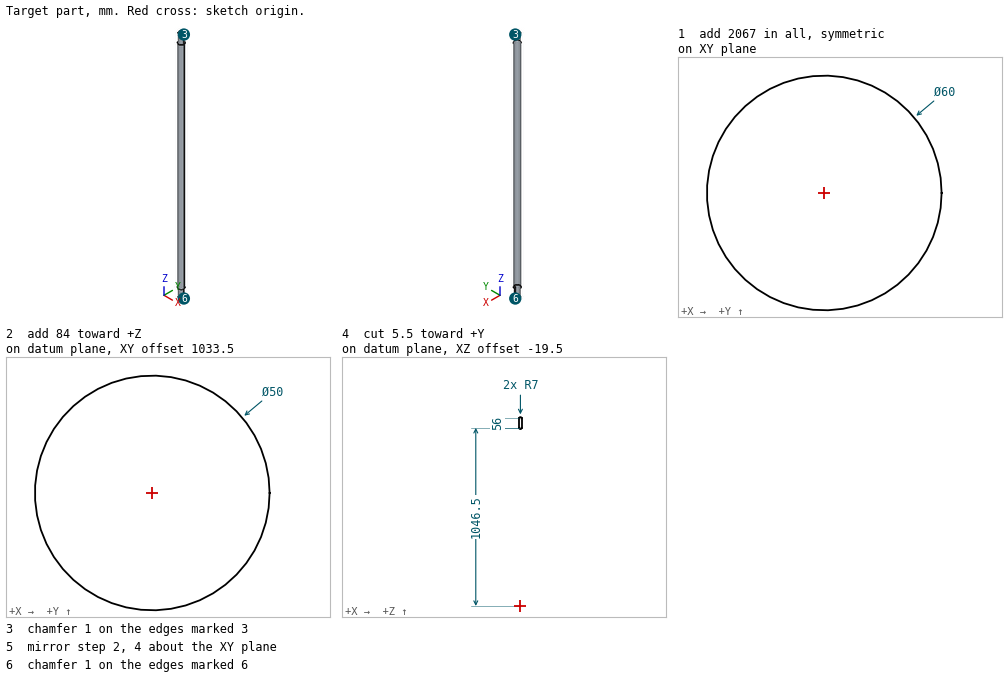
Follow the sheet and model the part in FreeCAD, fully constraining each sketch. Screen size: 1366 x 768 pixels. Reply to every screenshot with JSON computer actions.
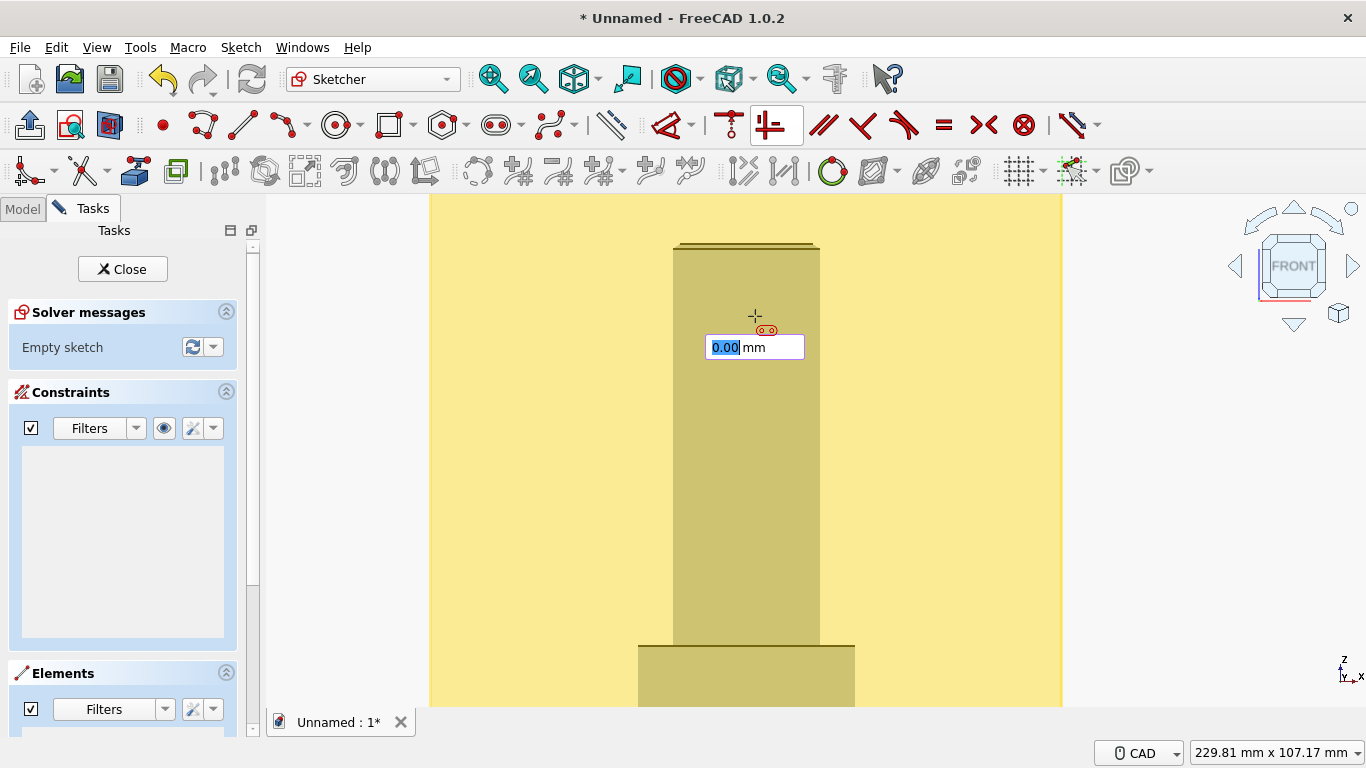
{"action": "left_click", "coordinate": [713, 450]}
{"action": "key", "text": "Escape"}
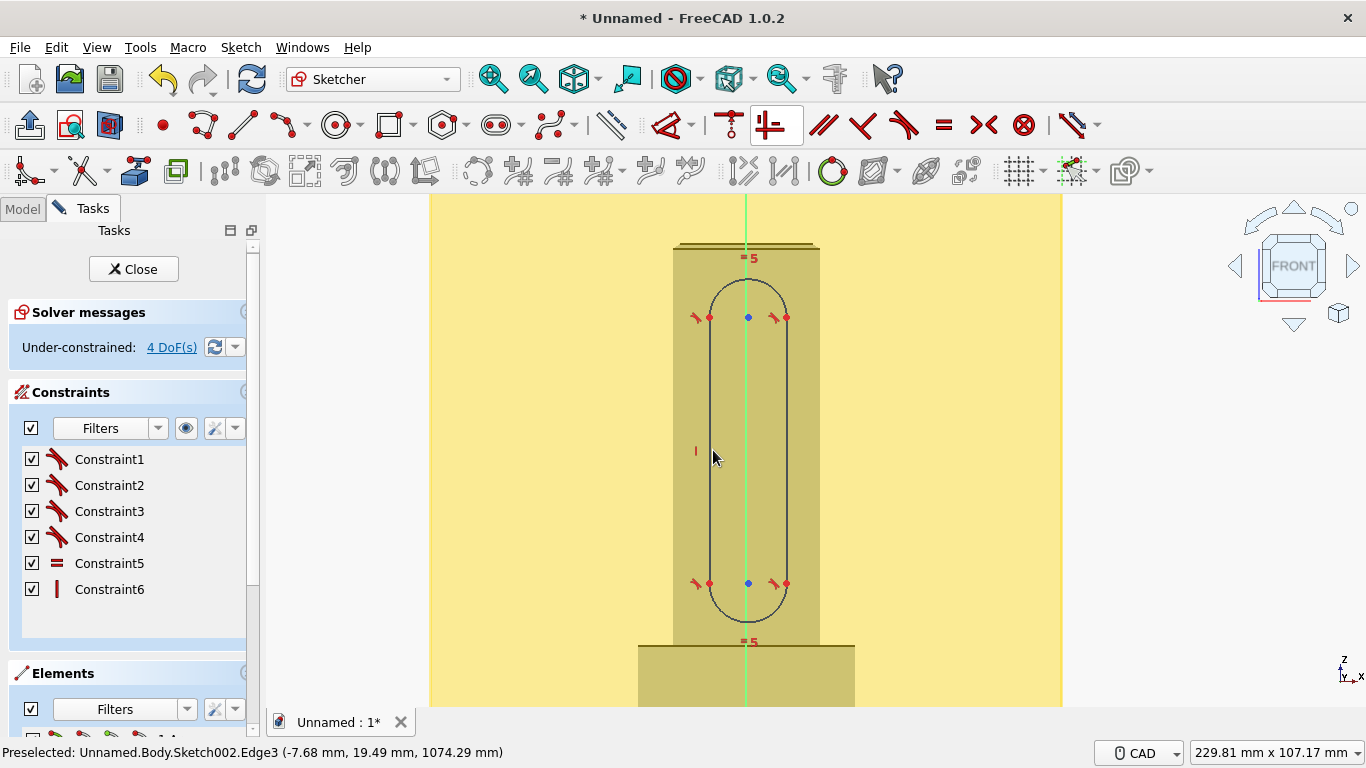
{"action": "left_click", "coordinate": [748, 584]}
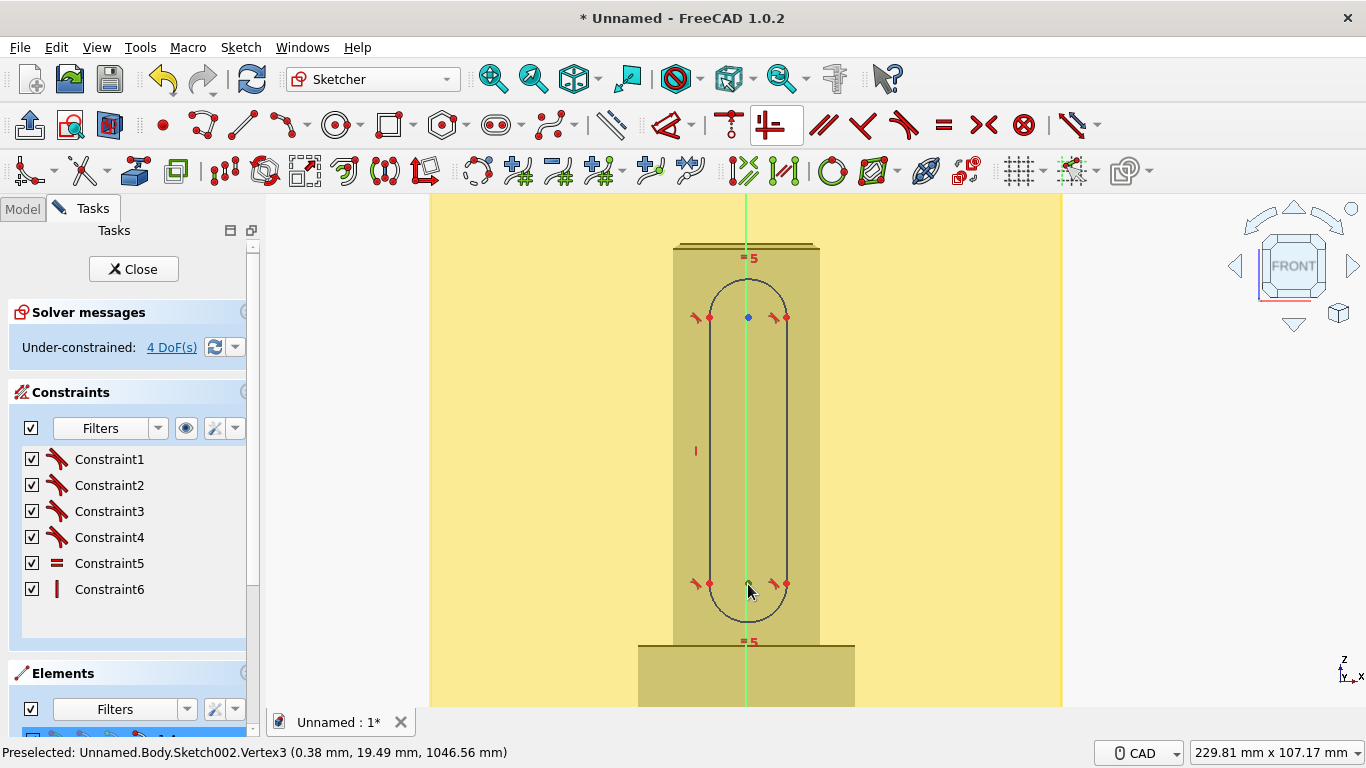
{"action": "left_click", "coordinate": [746, 548]}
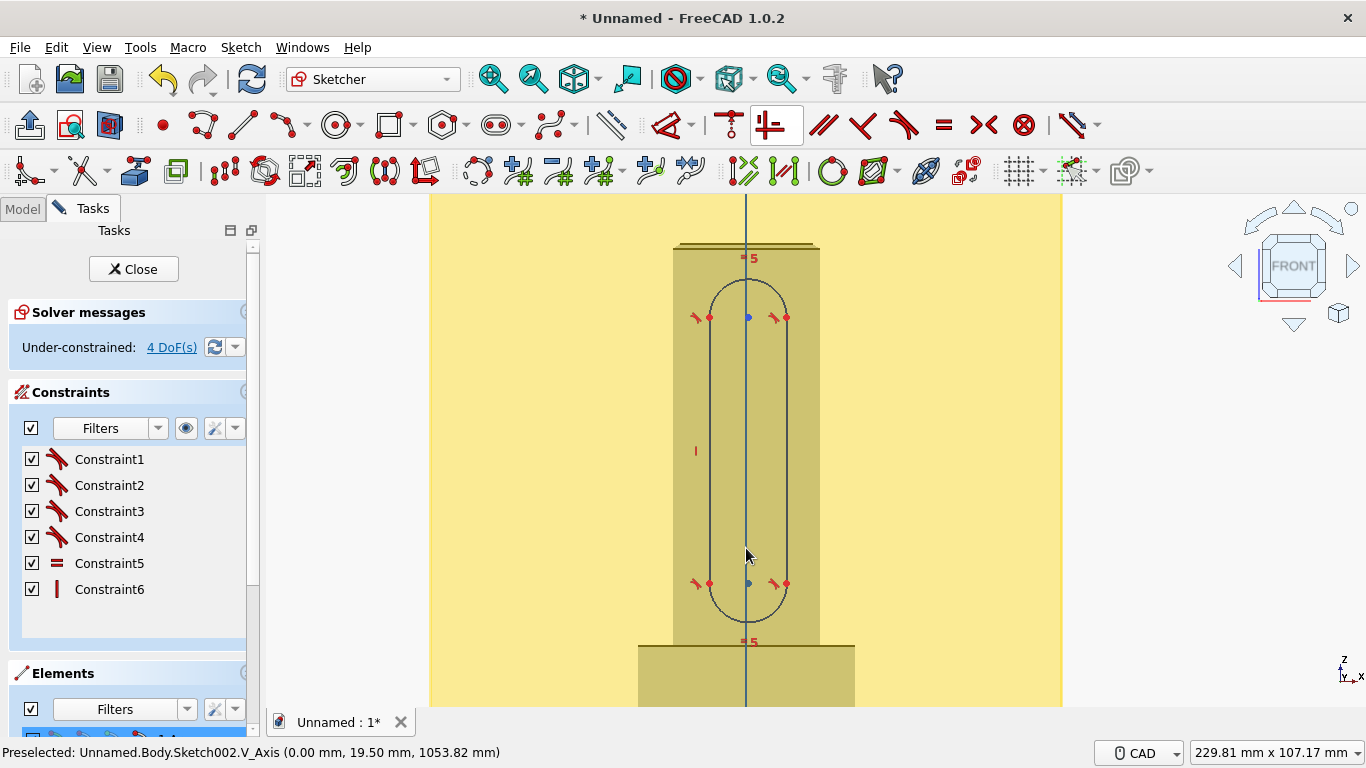
{"action": "left_click", "coordinate": [730, 126]}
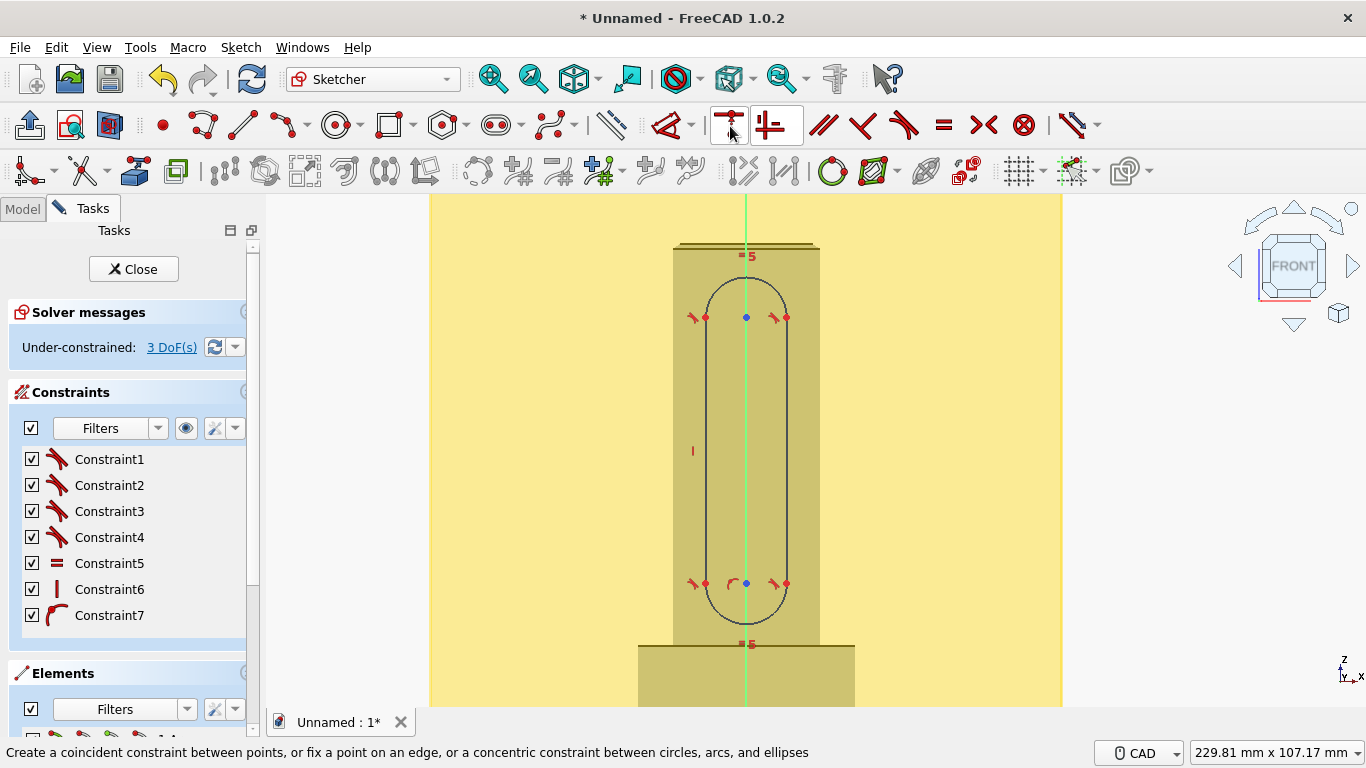
{"action": "left_click", "coordinate": [666, 126]}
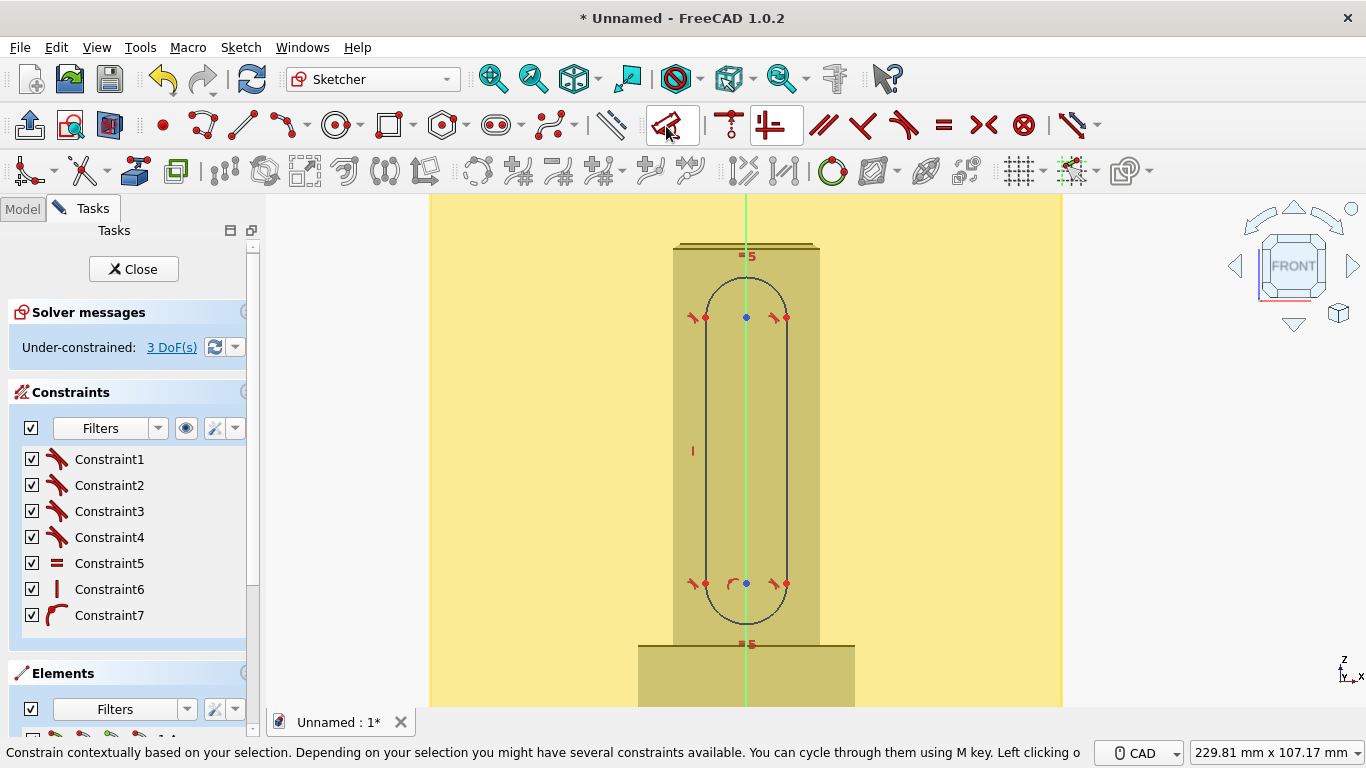
{"action": "left_click", "coordinate": [723, 616]}
{"action": "left_click", "coordinate": [704, 642]}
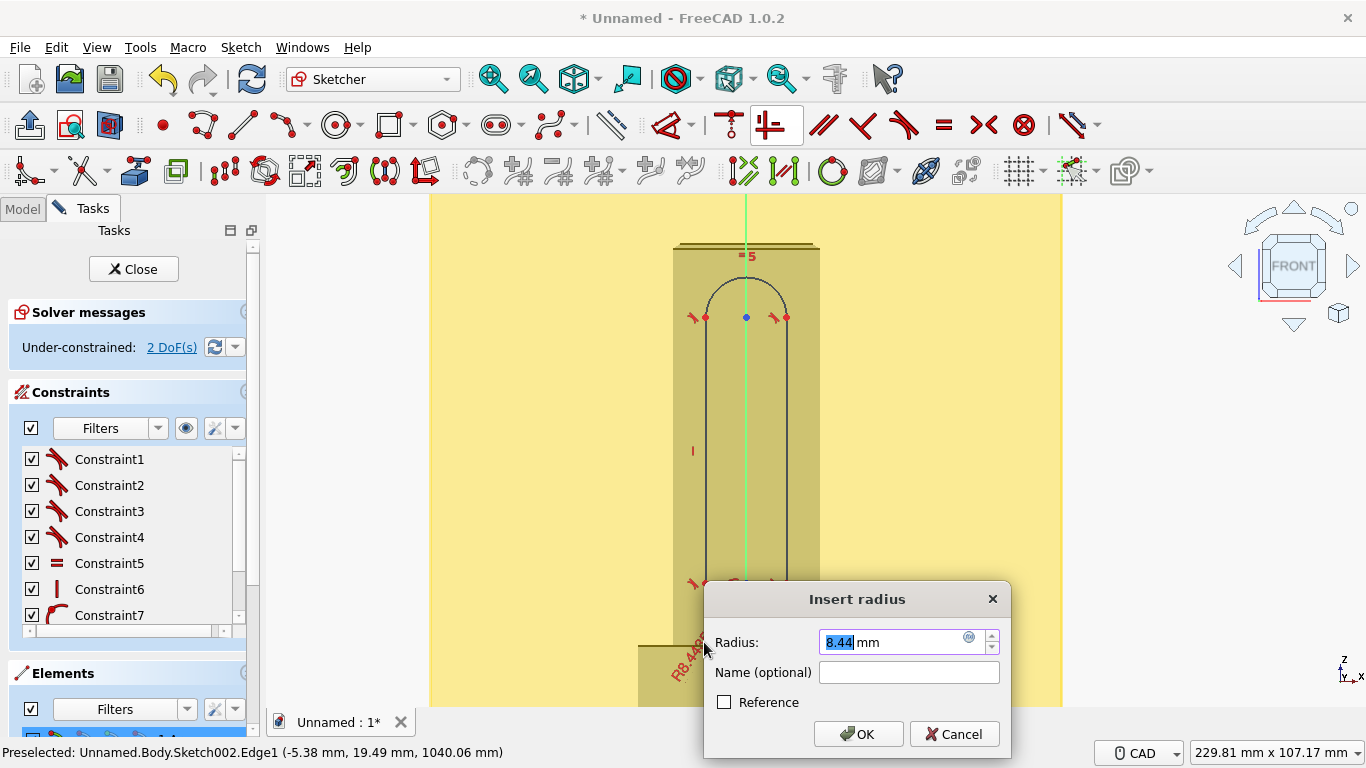
{"action": "type", "text": "7"}
{"action": "key", "text": "Return"}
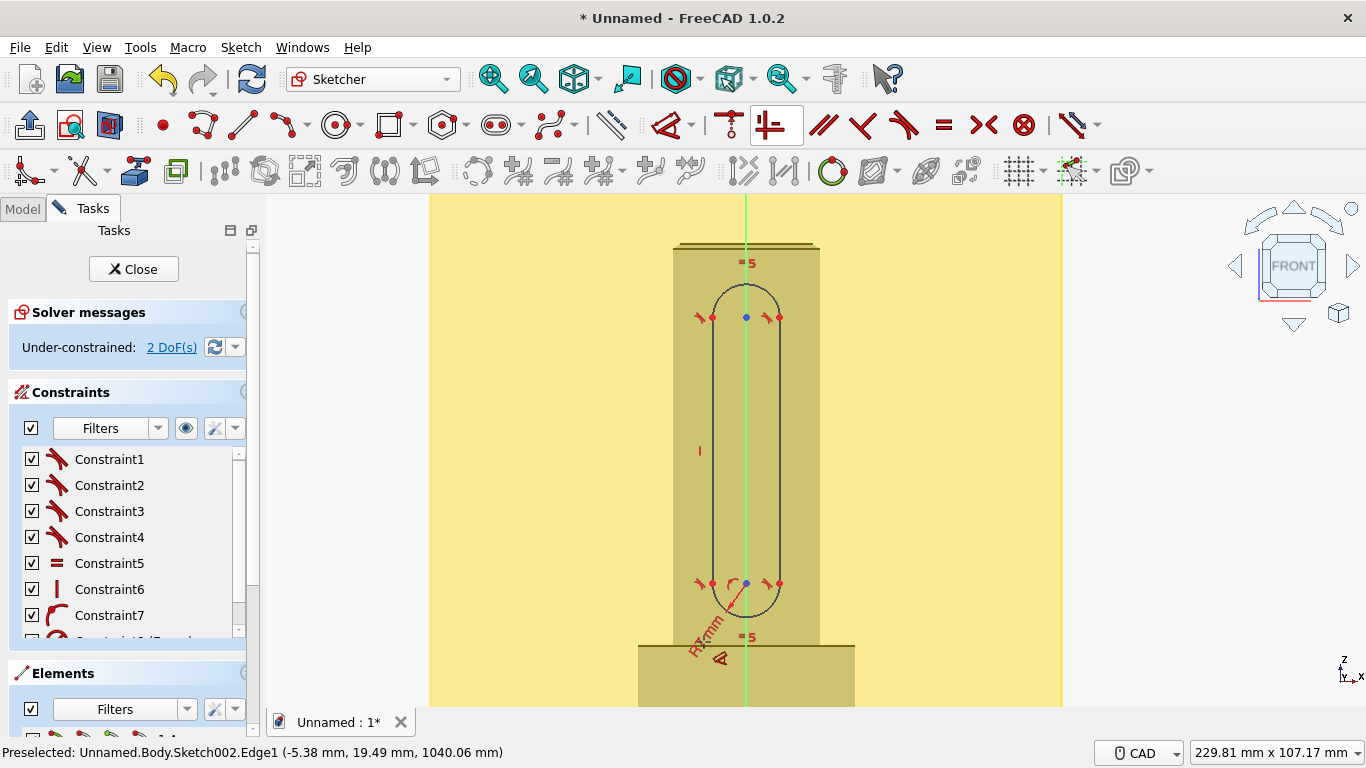
{"action": "left_click", "coordinate": [713, 504]}
{"action": "left_click", "coordinate": [679, 451]}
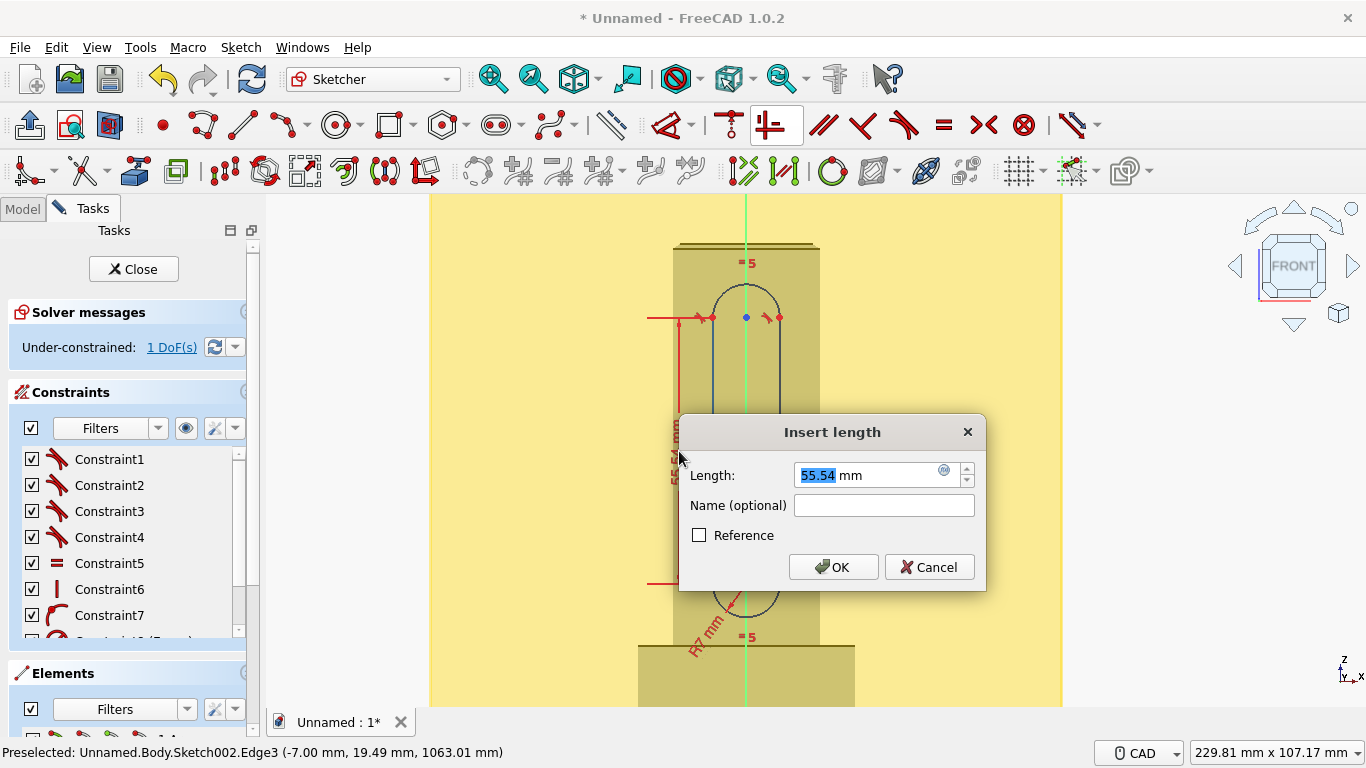
{"action": "type", "text": "56"}
{"action": "key", "text": "Return"}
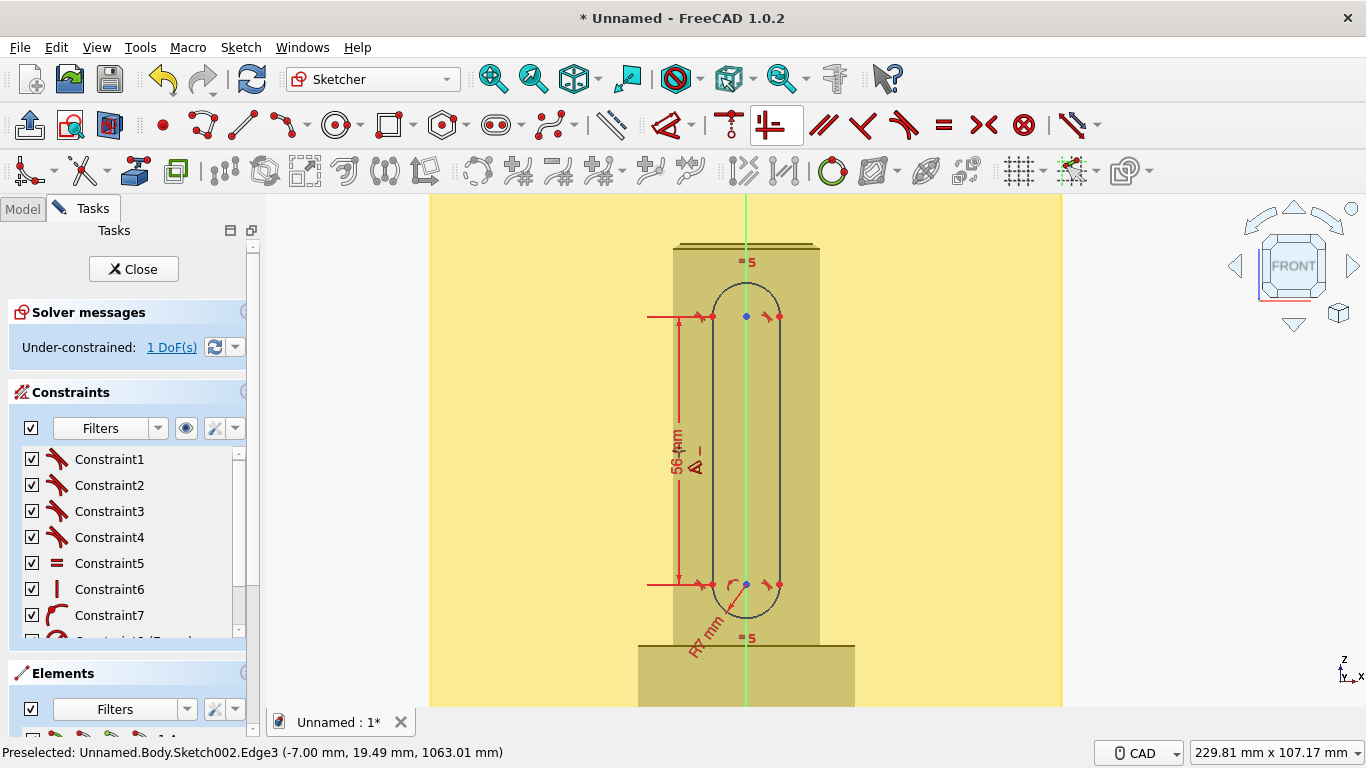
{"action": "left_click", "coordinate": [713, 585]}
{"action": "left_click", "coordinate": [679, 610]}